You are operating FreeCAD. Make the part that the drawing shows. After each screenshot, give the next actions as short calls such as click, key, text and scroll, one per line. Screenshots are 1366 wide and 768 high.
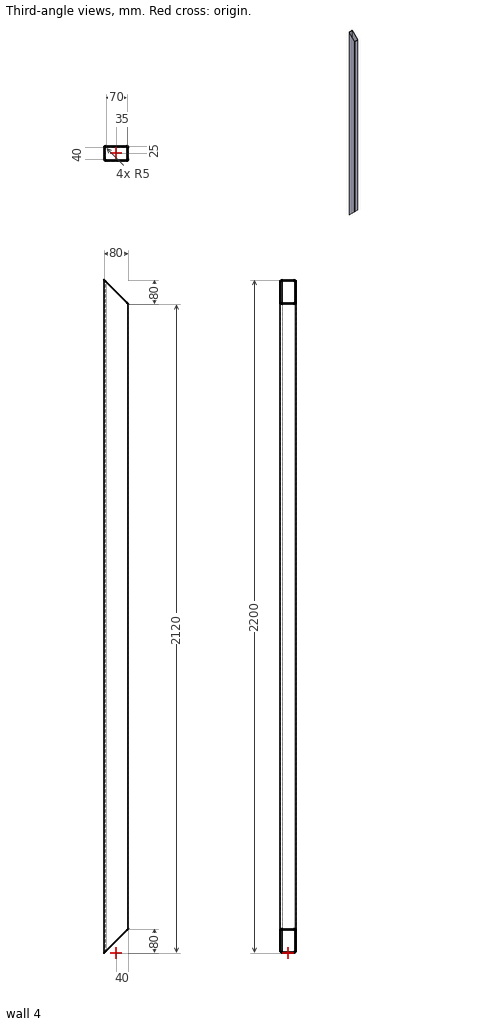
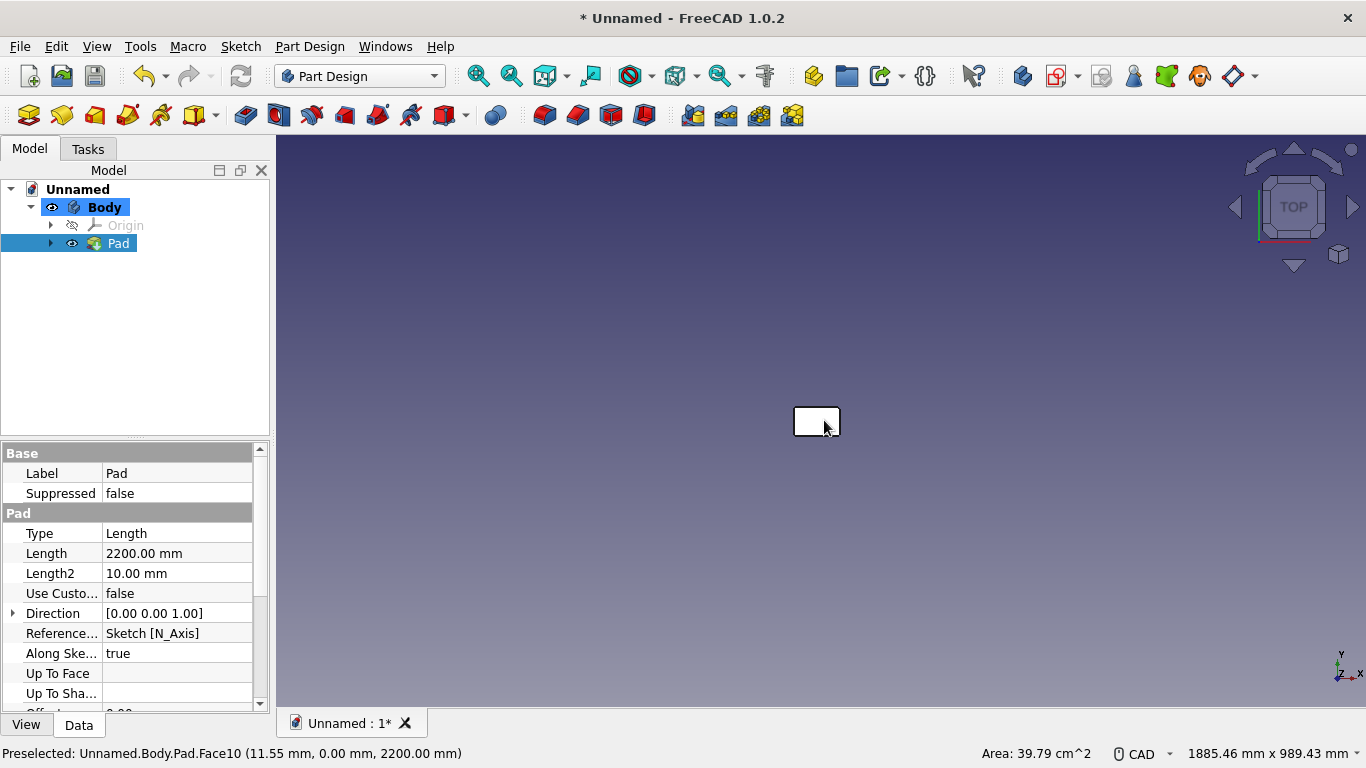
click(479, 76)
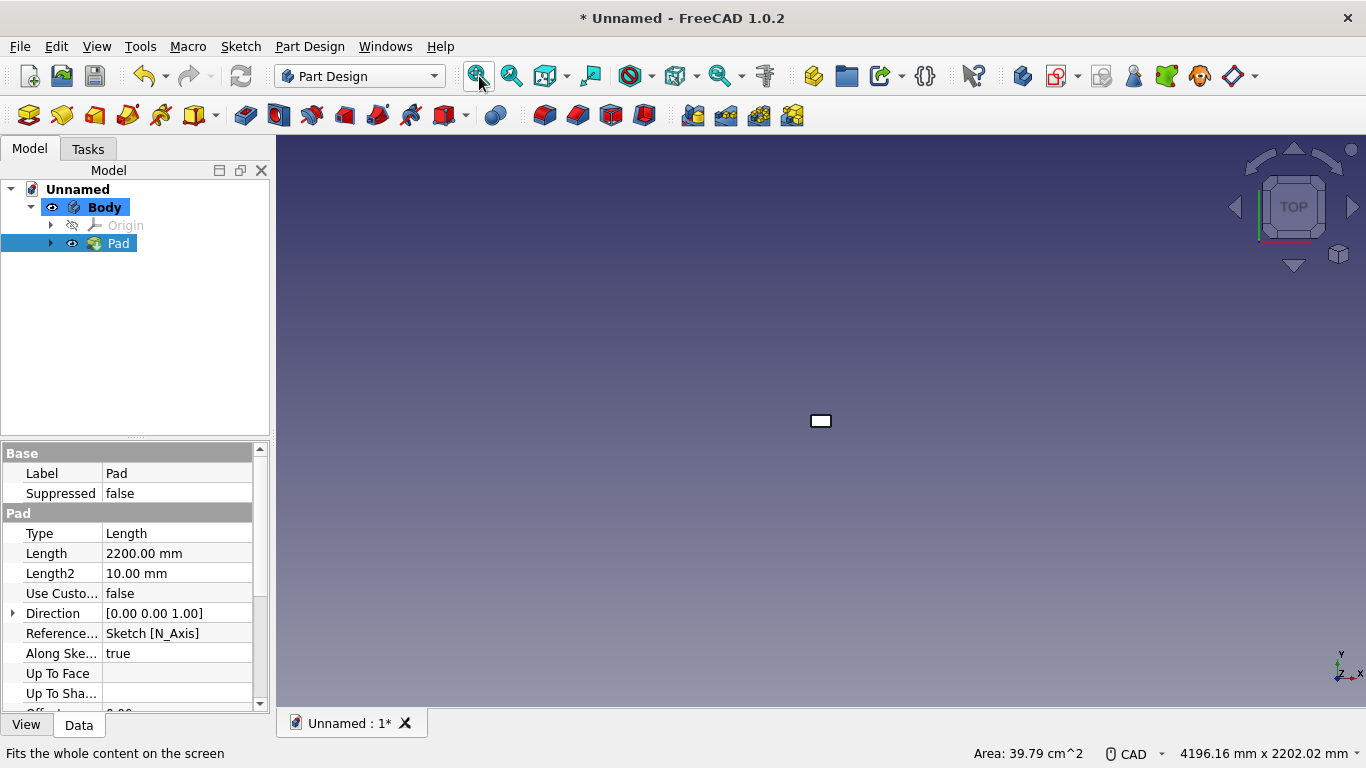
key(1)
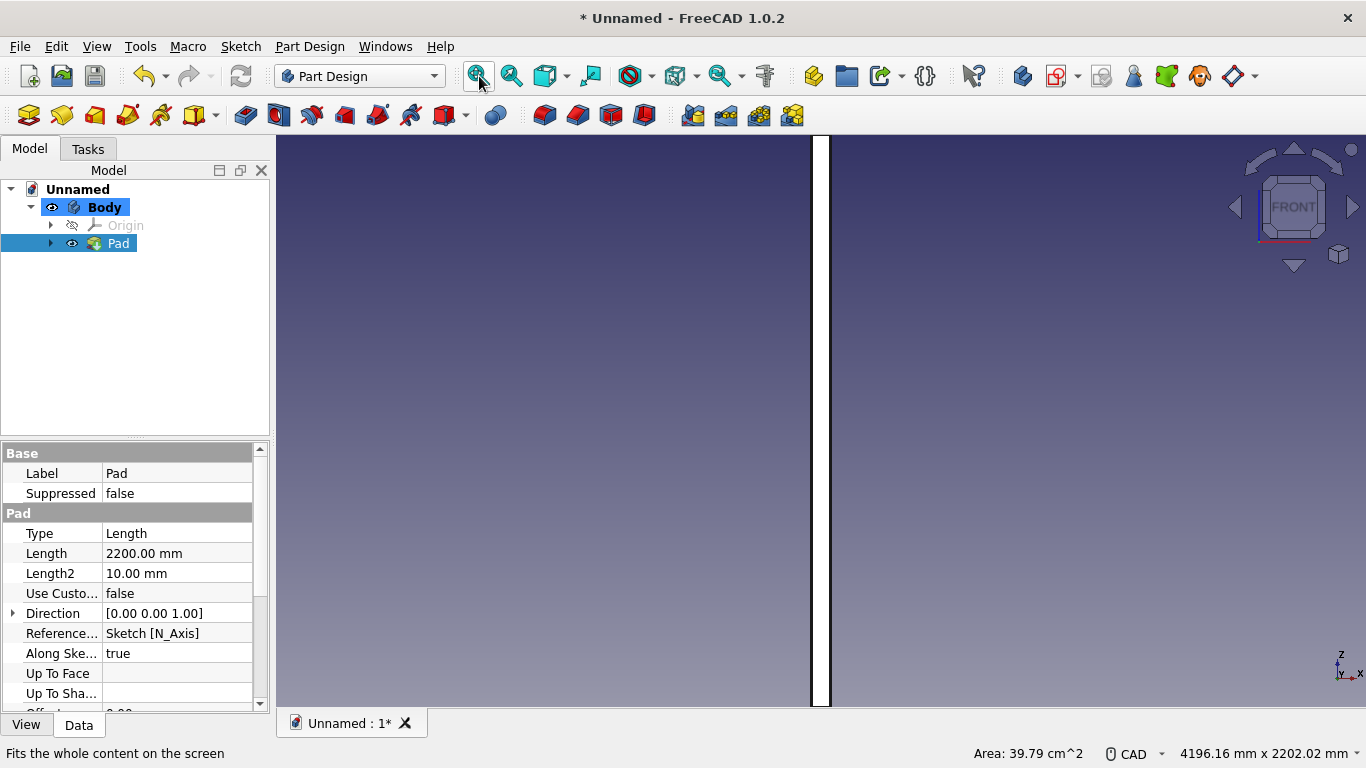
click(479, 76)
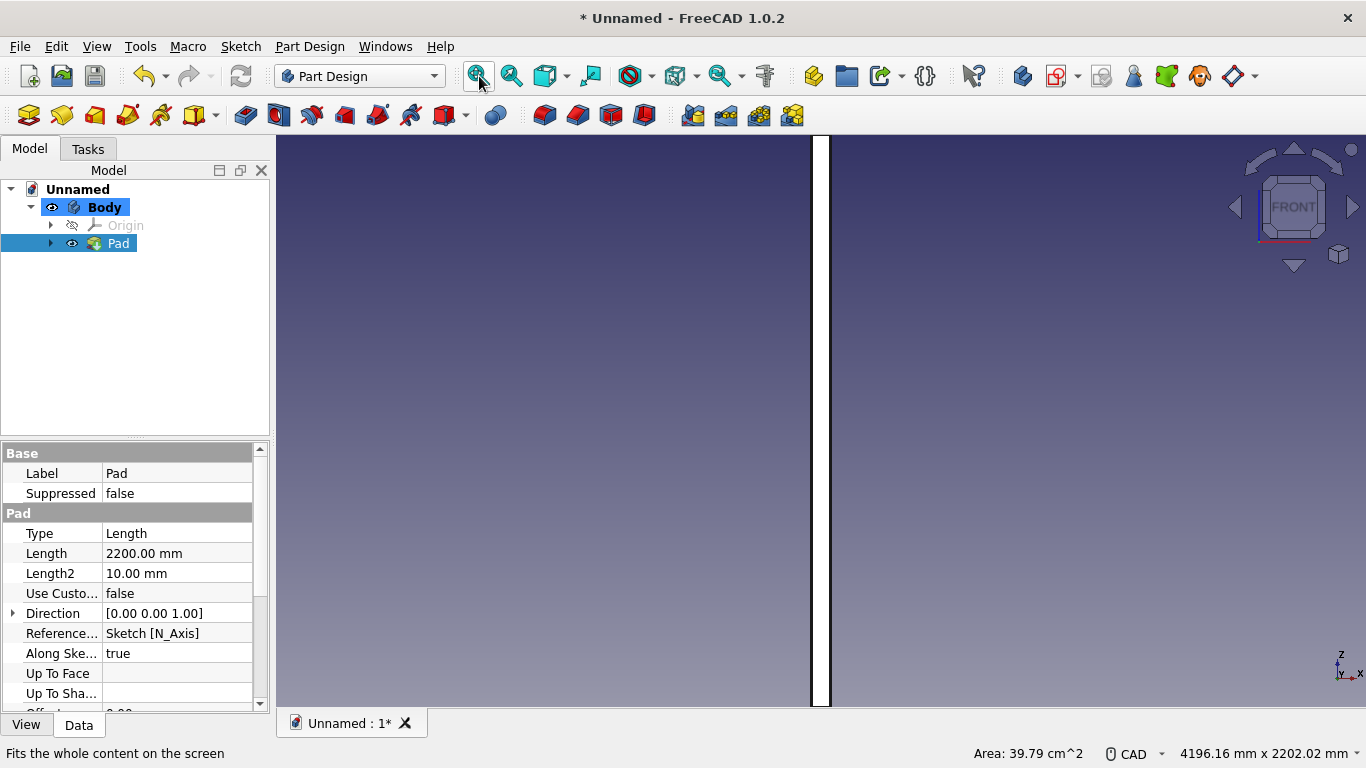
key(3)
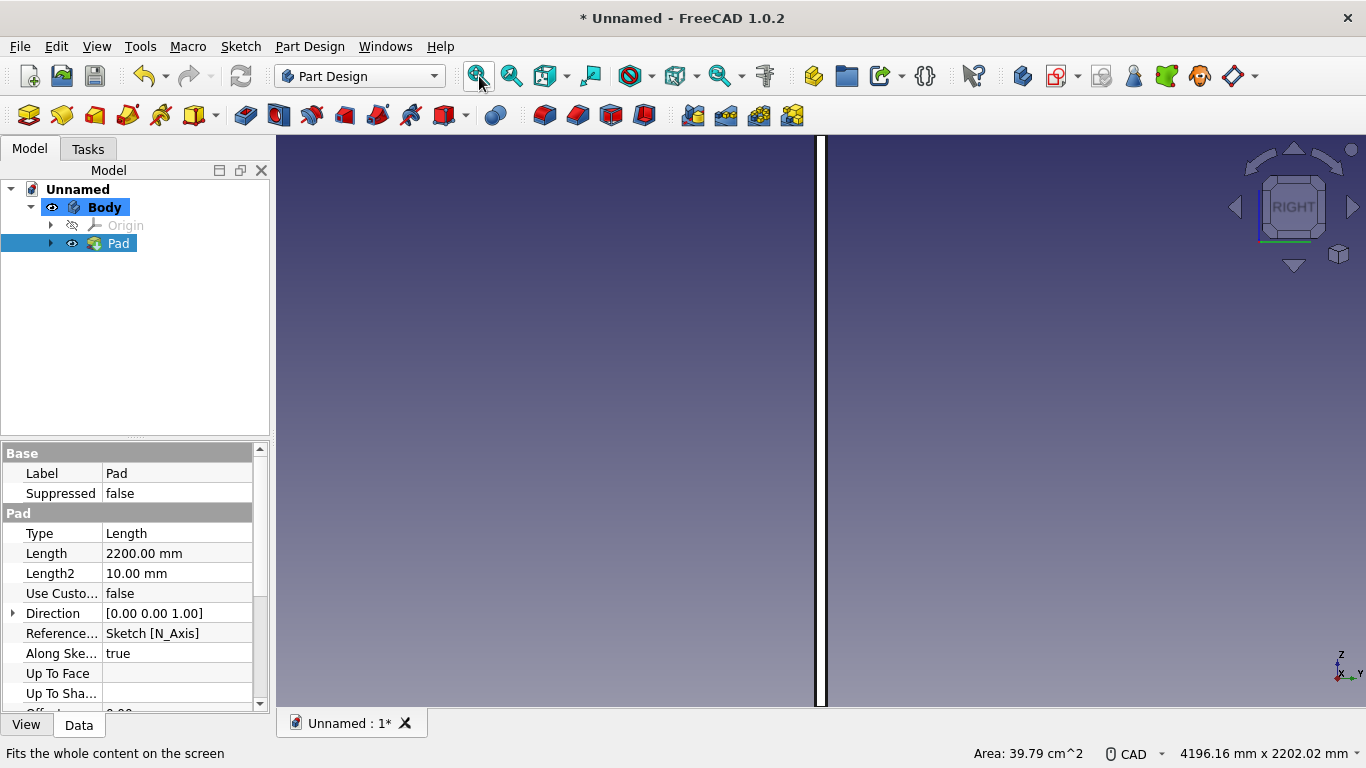
click(479, 76)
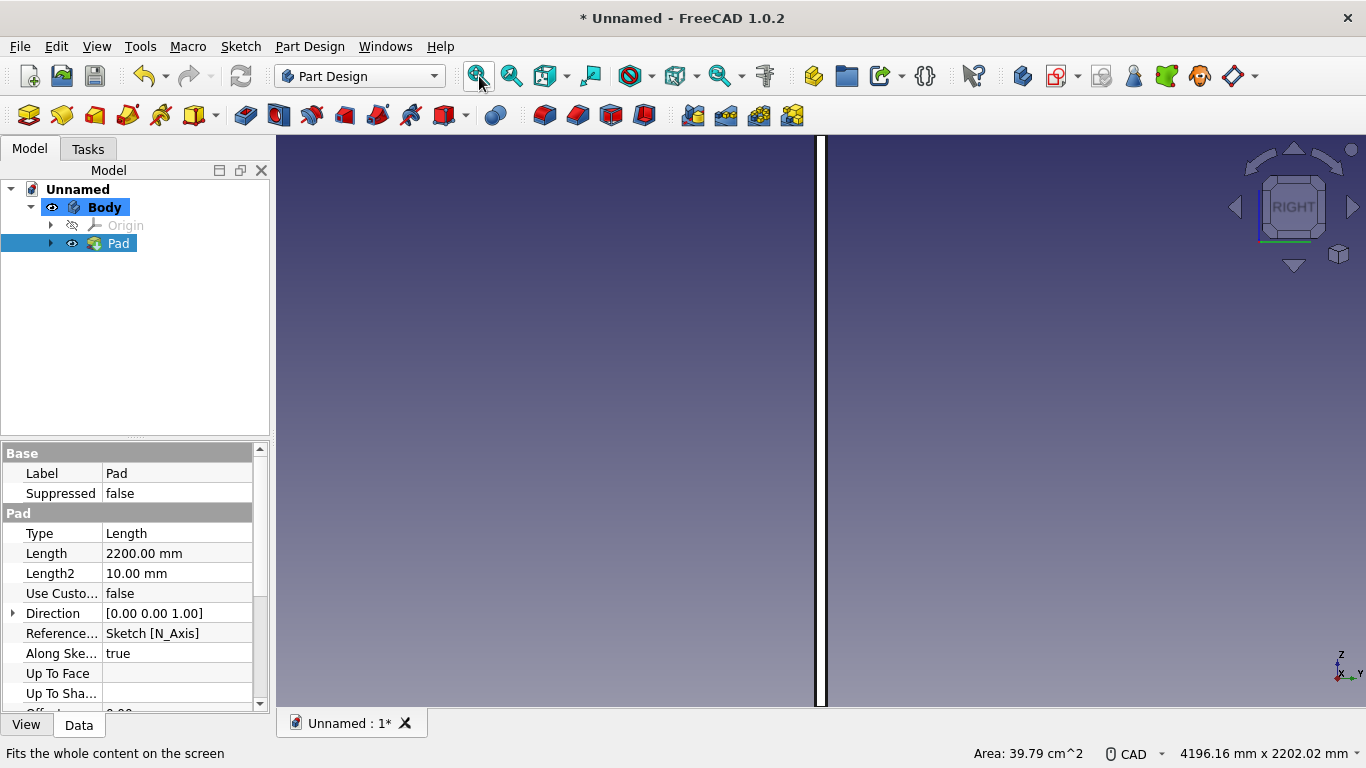
key(5)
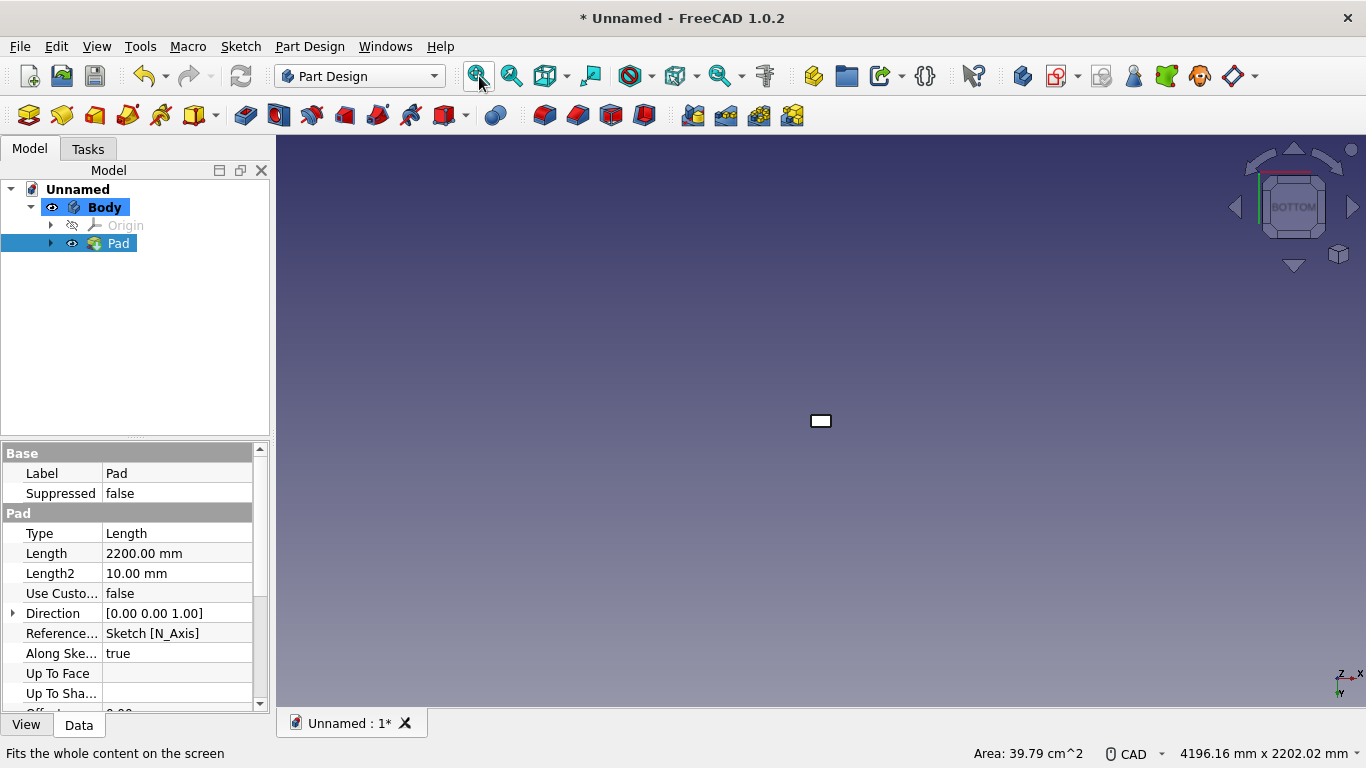
click(479, 76)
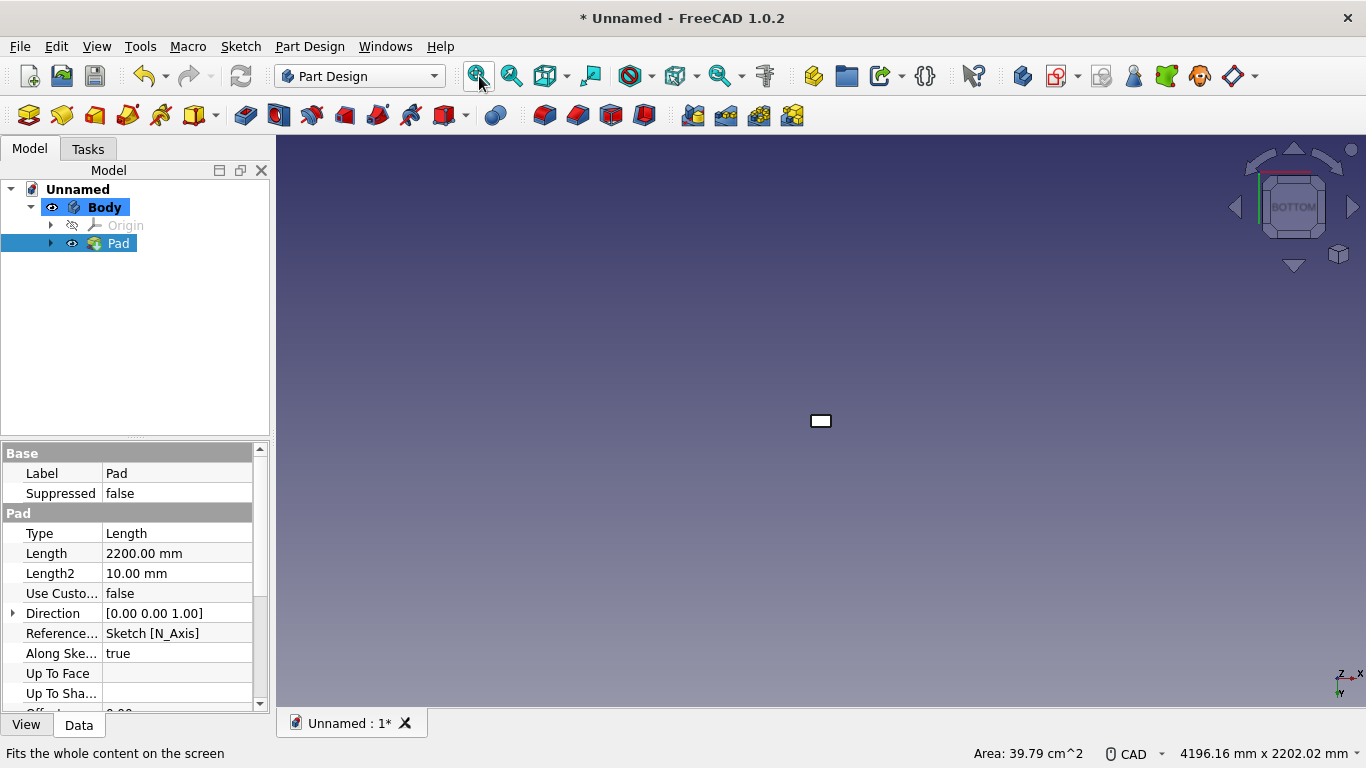
scroll(824, 420, up, 4)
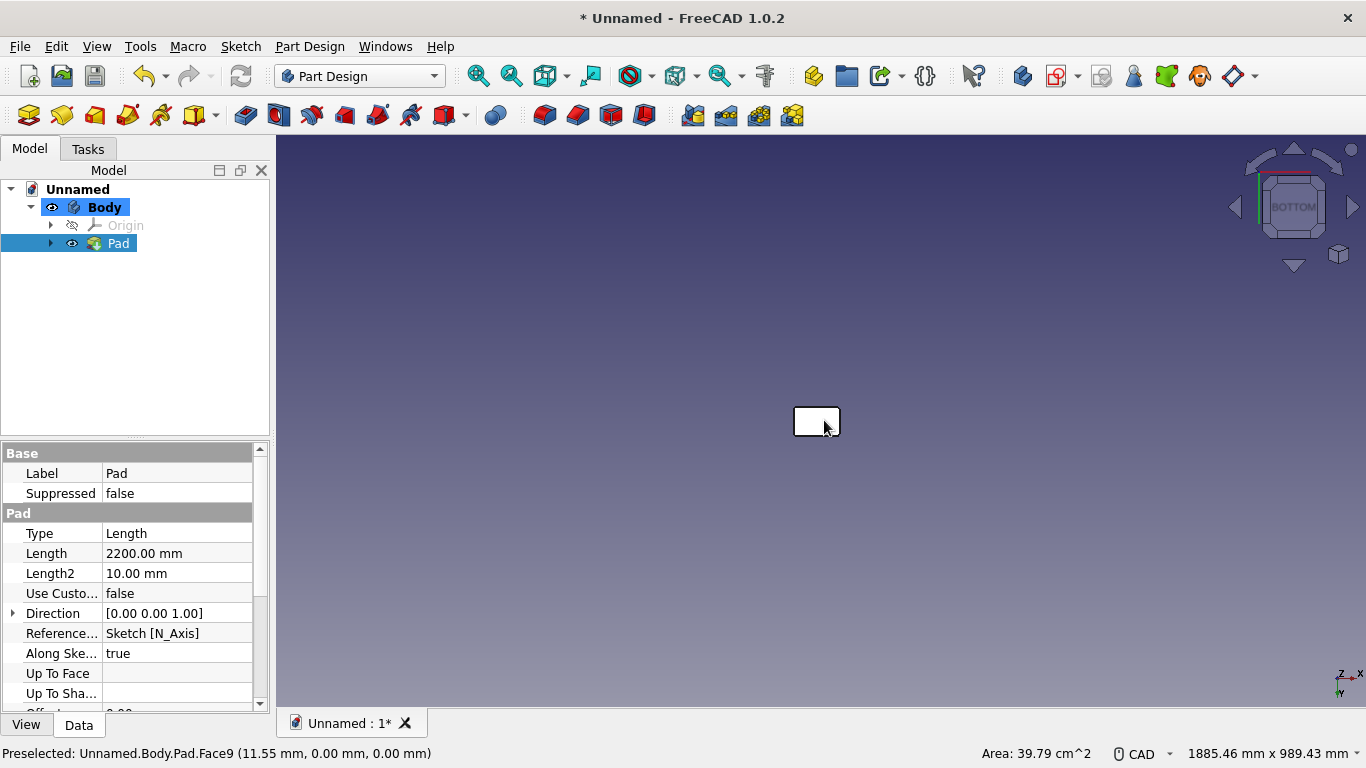
click(823, 421, ctrl)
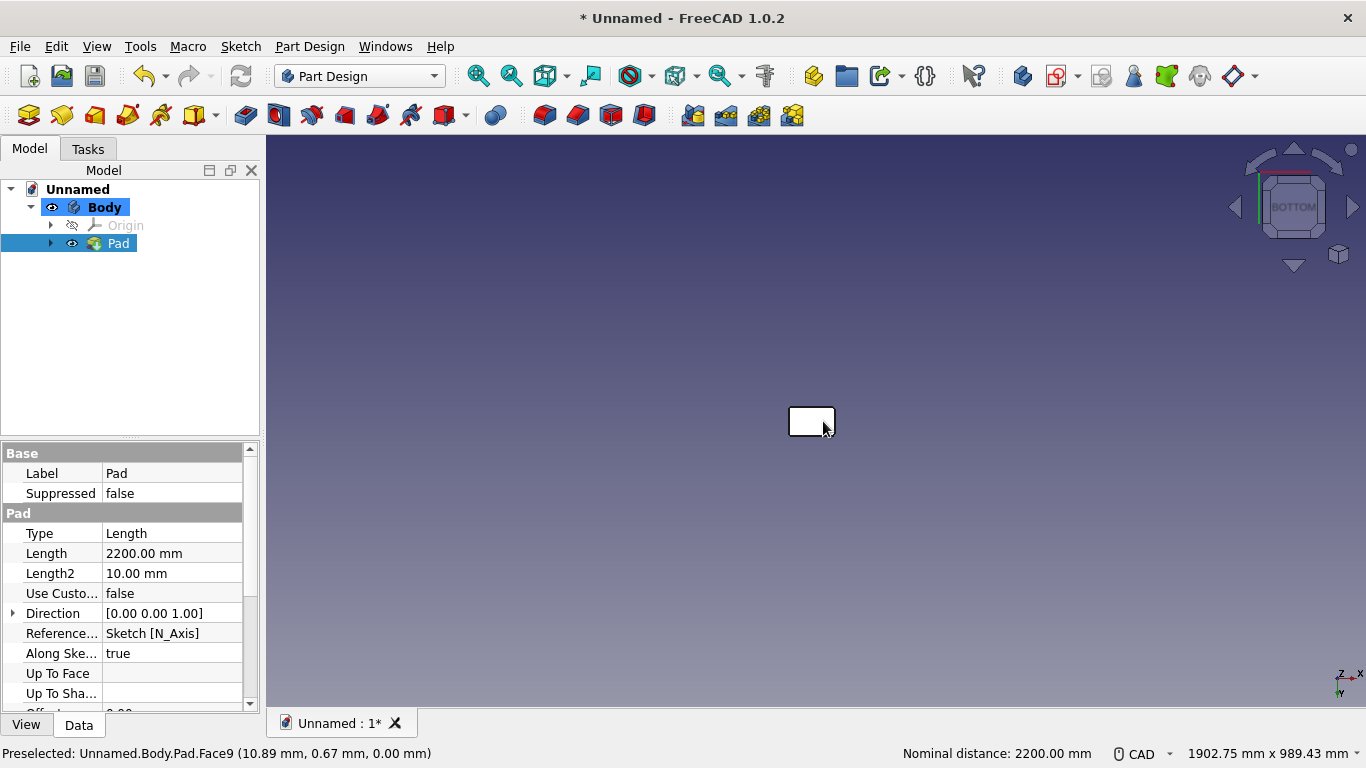
click(644, 116)